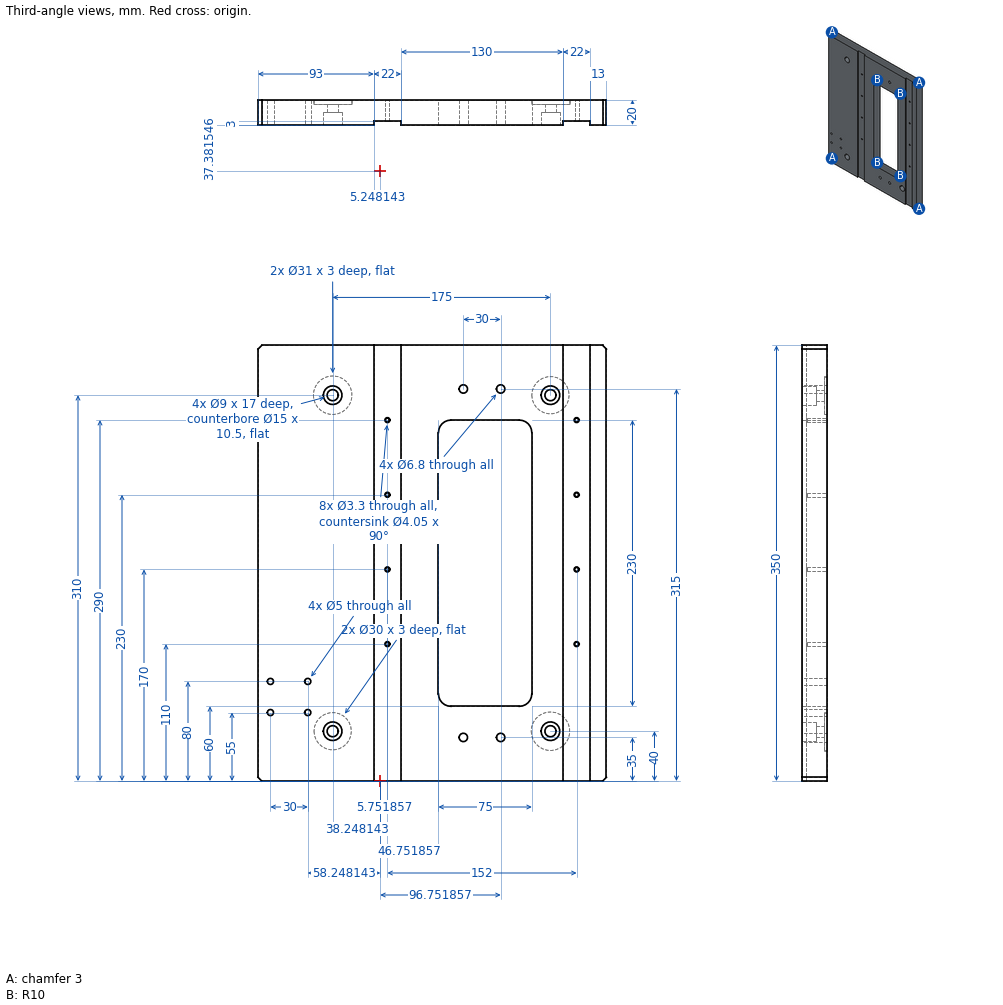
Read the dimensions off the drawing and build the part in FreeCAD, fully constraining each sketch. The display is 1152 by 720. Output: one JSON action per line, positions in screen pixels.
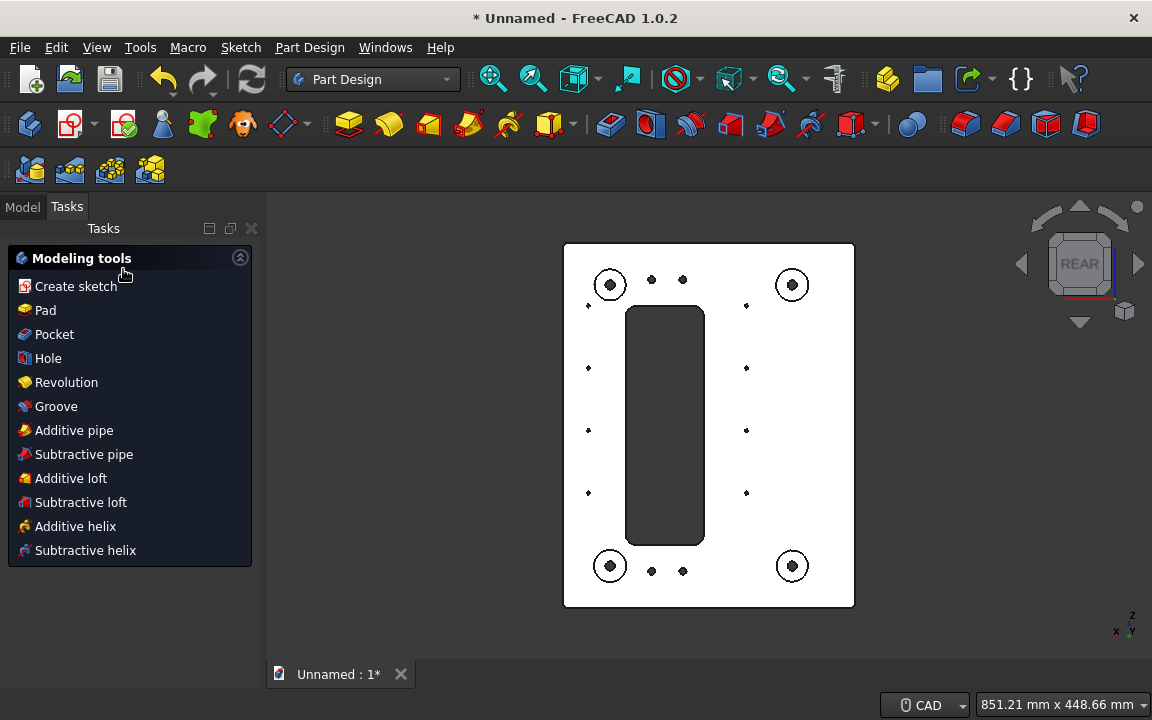
{"action": "left_click", "coordinate": [652, 124]}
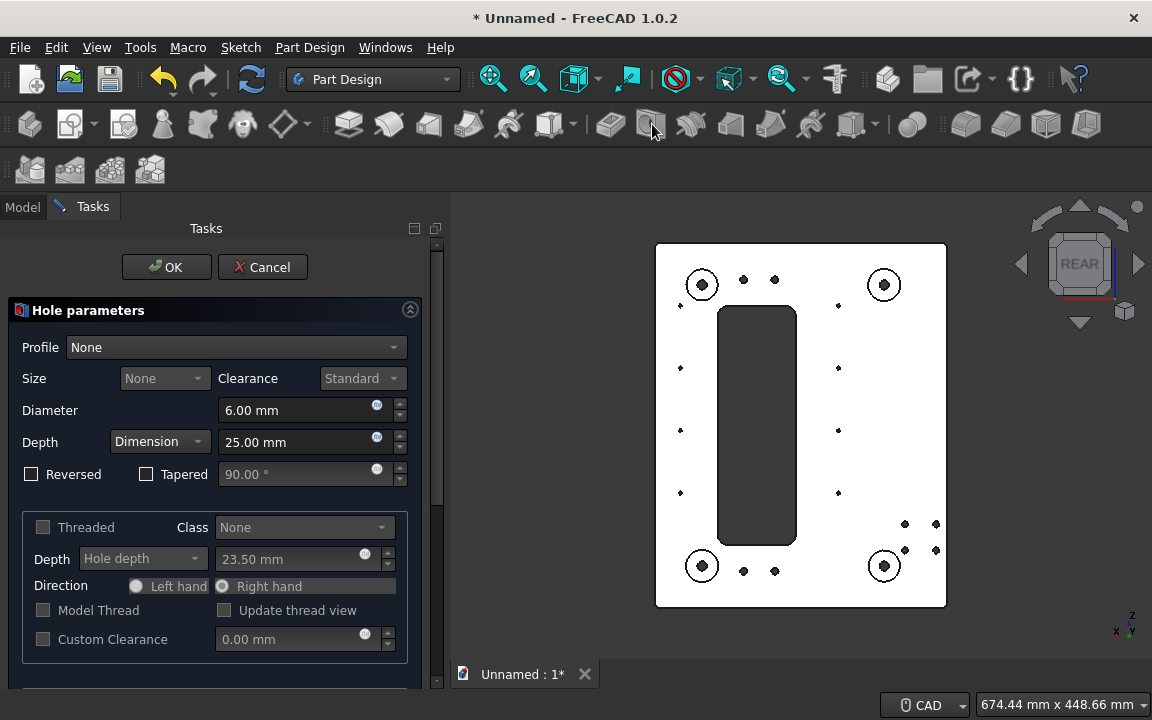
{"action": "triple_click", "coordinate": [305, 410]}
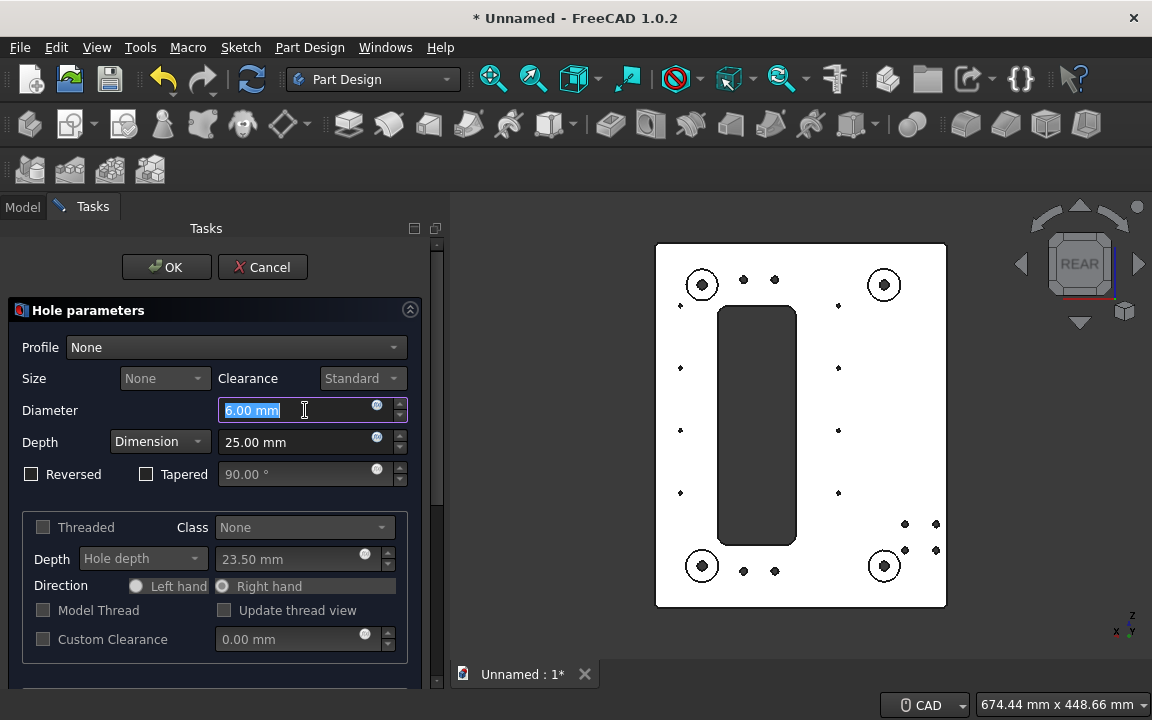
{"action": "type", "text": "5"}
{"action": "key", "text": "Tab"}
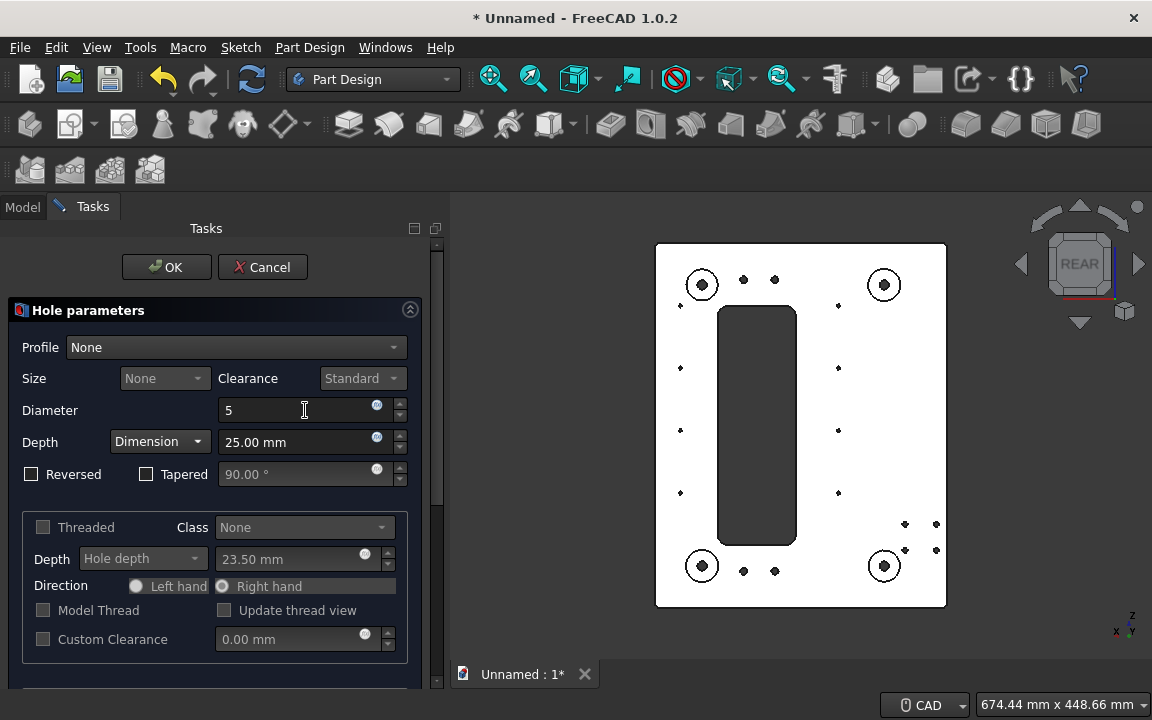
{"action": "left_click", "coordinate": [161, 442]}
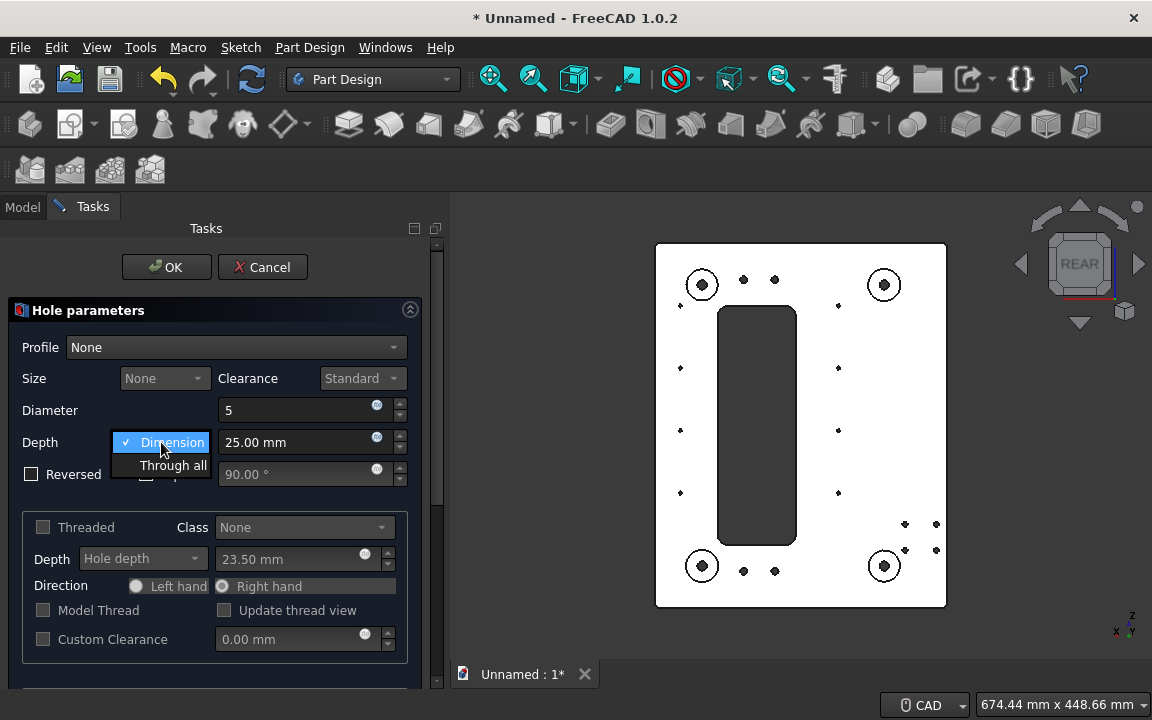
{"action": "left_click", "coordinate": [160, 466]}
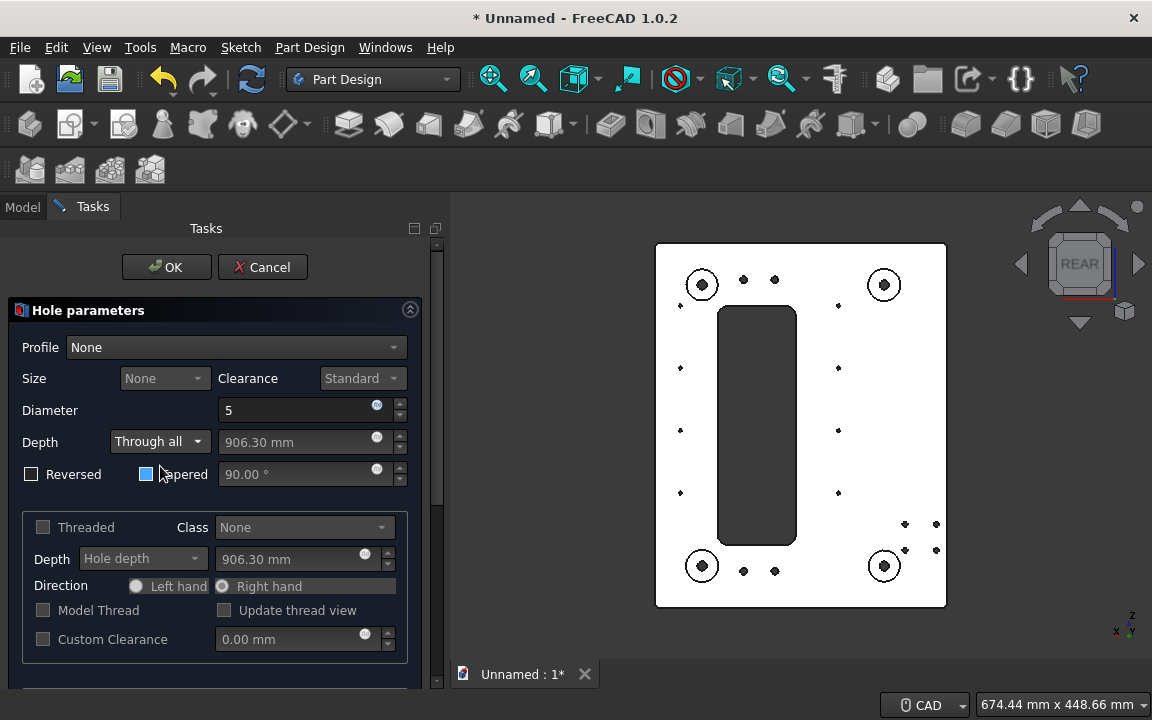
{"action": "left_click", "coordinate": [167, 267]}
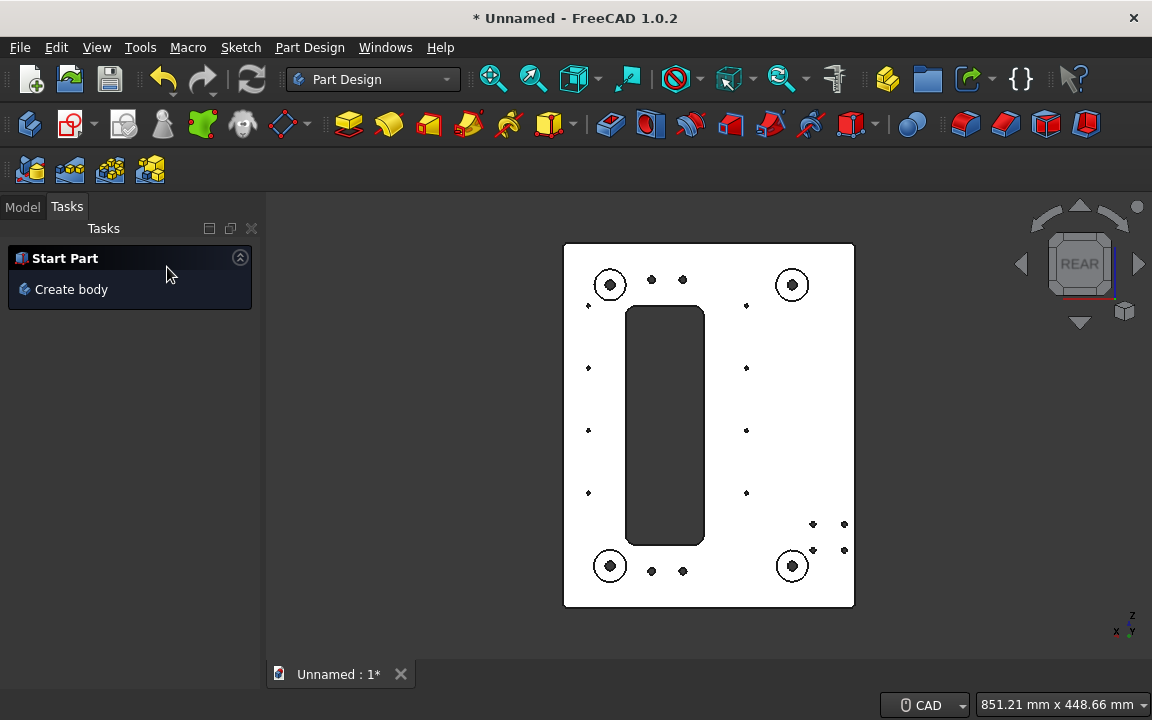
{"action": "key", "text": "0"}